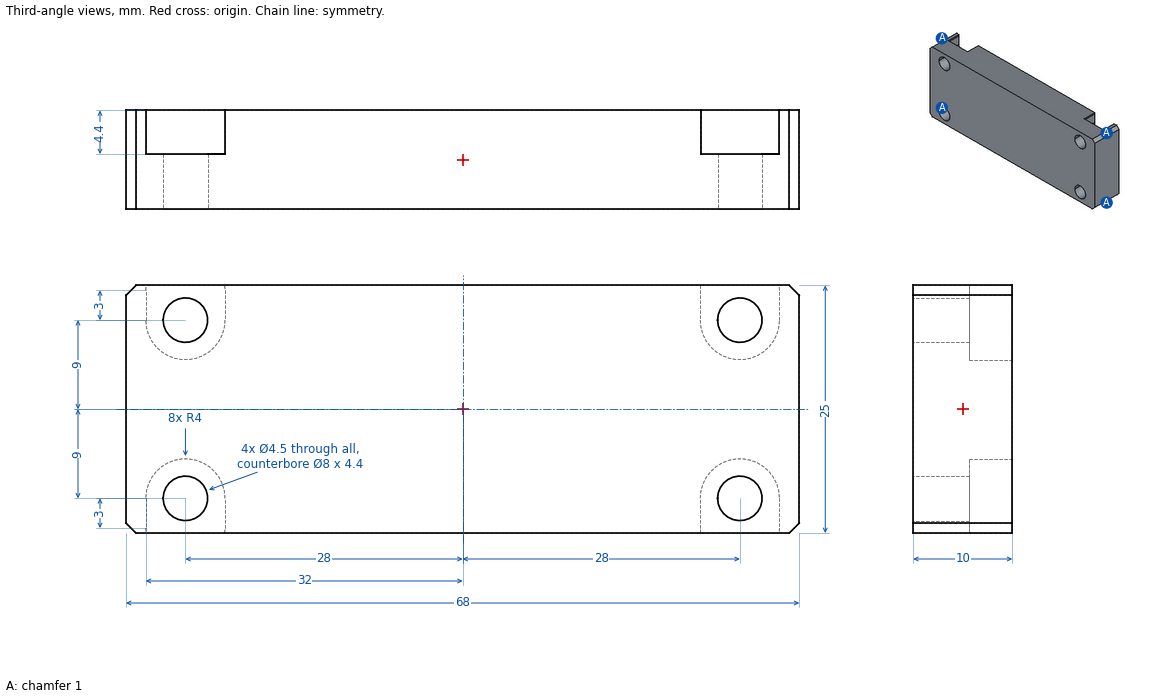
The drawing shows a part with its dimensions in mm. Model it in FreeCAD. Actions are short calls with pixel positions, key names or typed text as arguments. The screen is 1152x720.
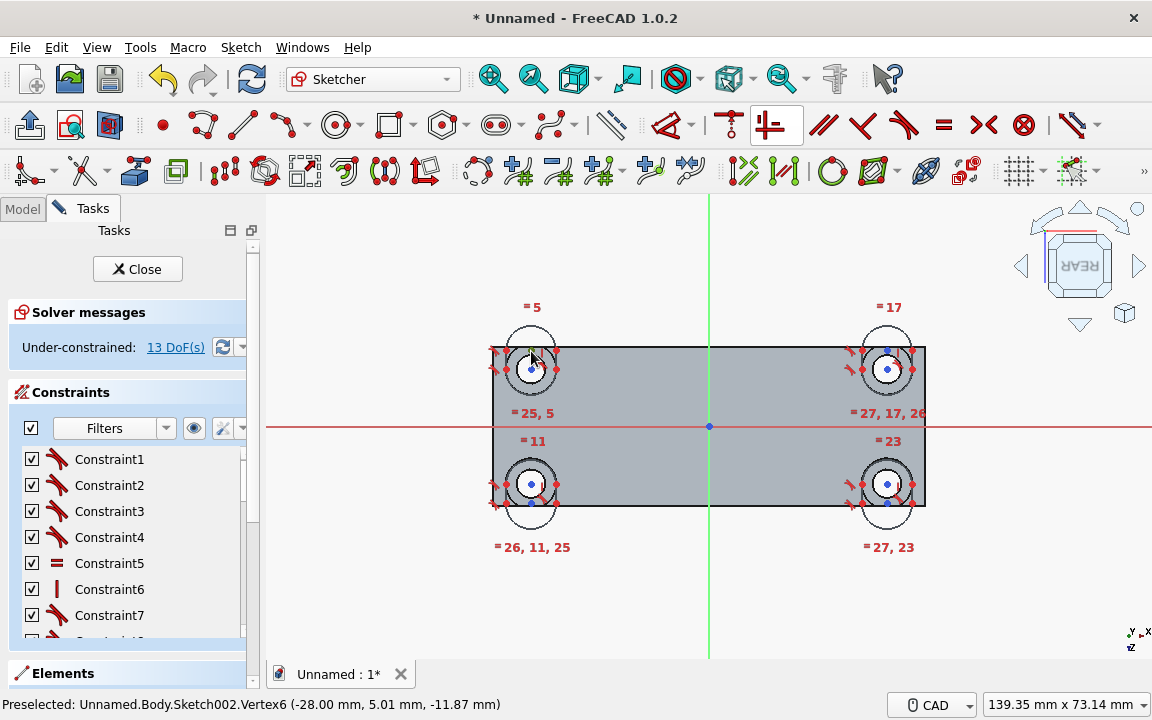
click(531, 504)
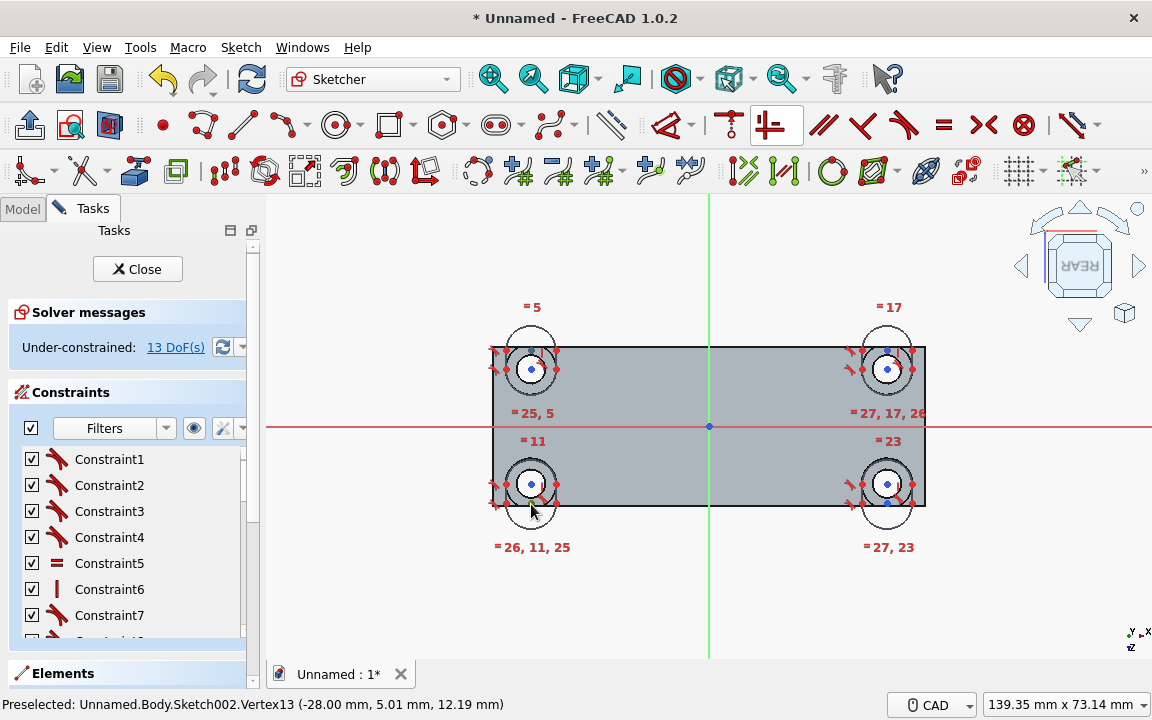
click(344, 426)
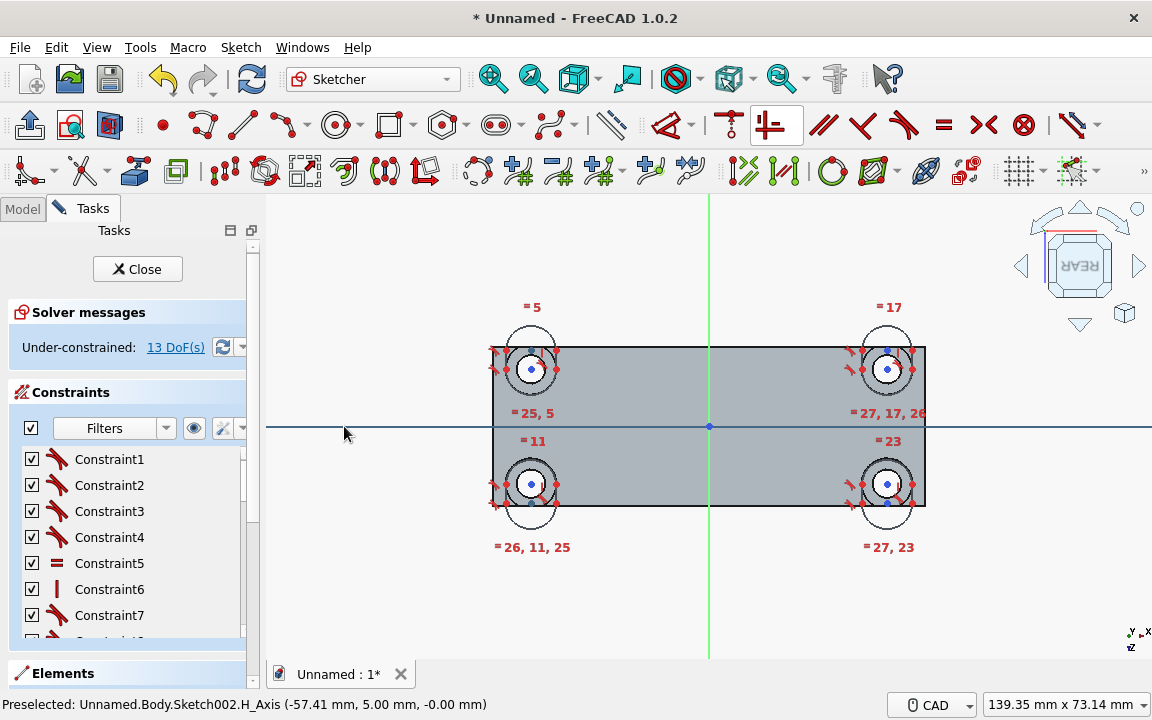
click(984, 126)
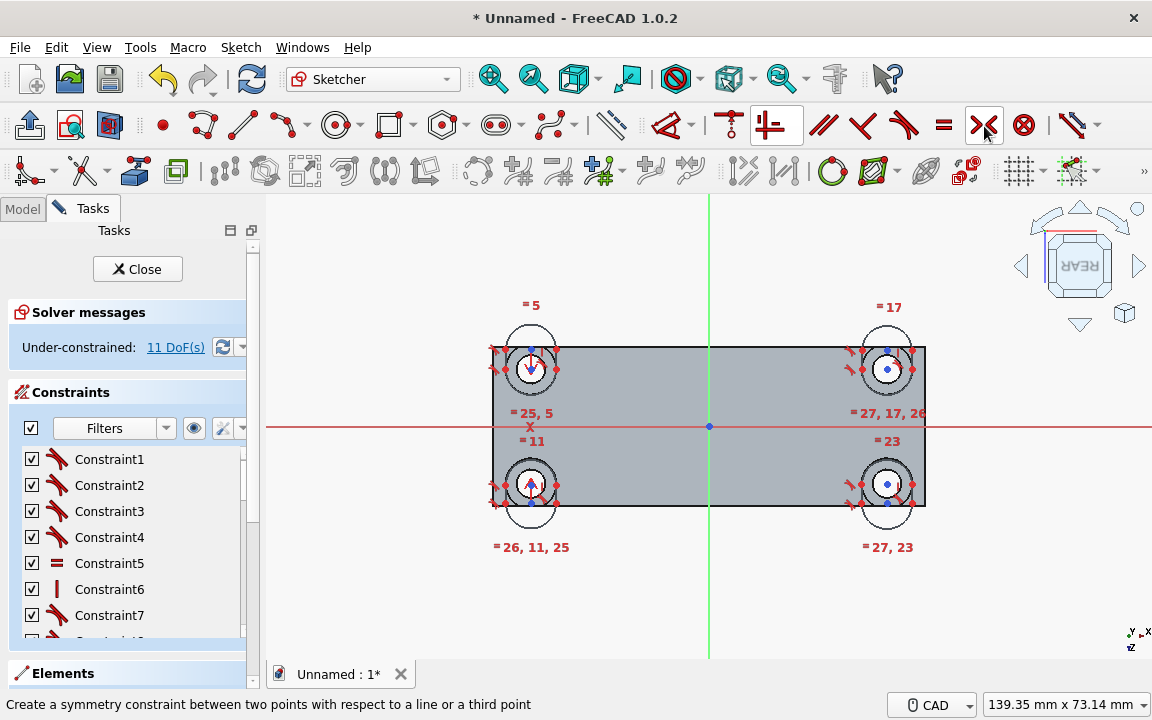
click(531, 370)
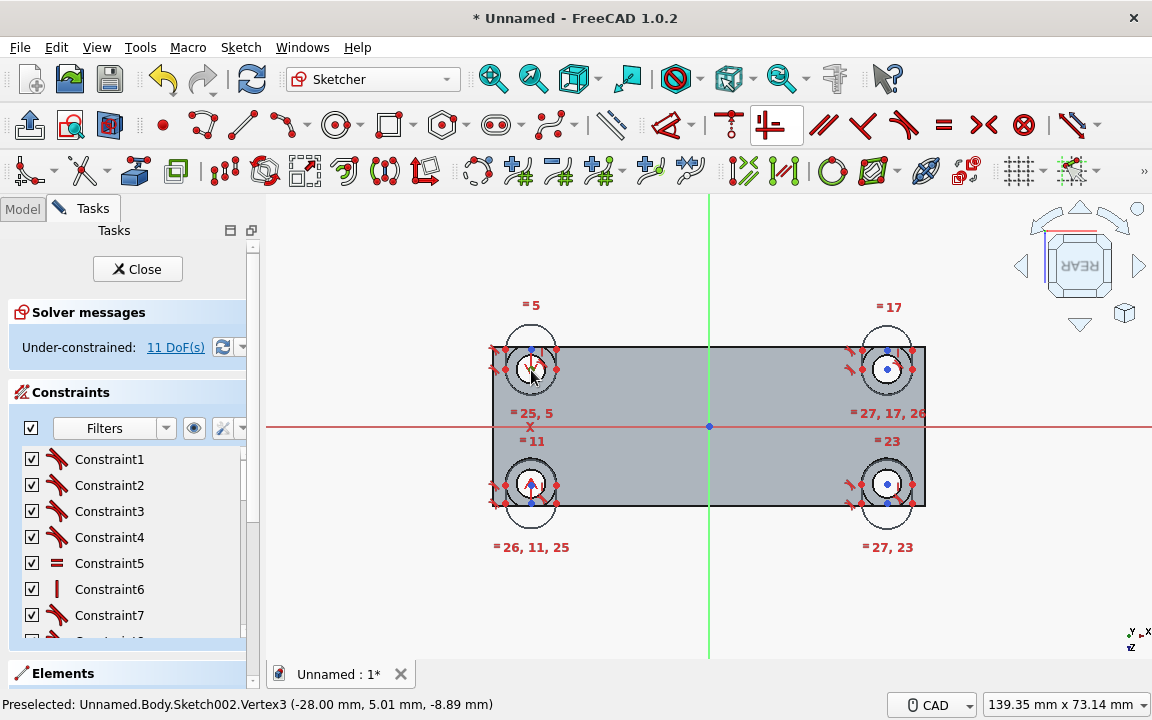
click(887, 370)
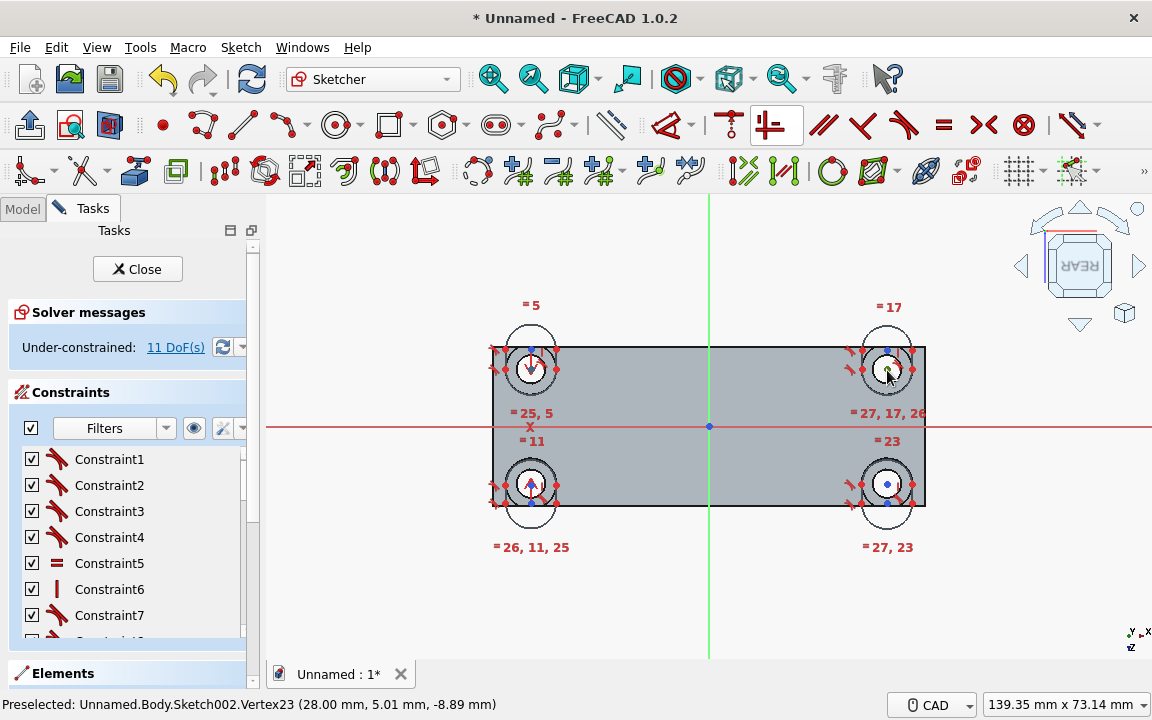
click(709, 602)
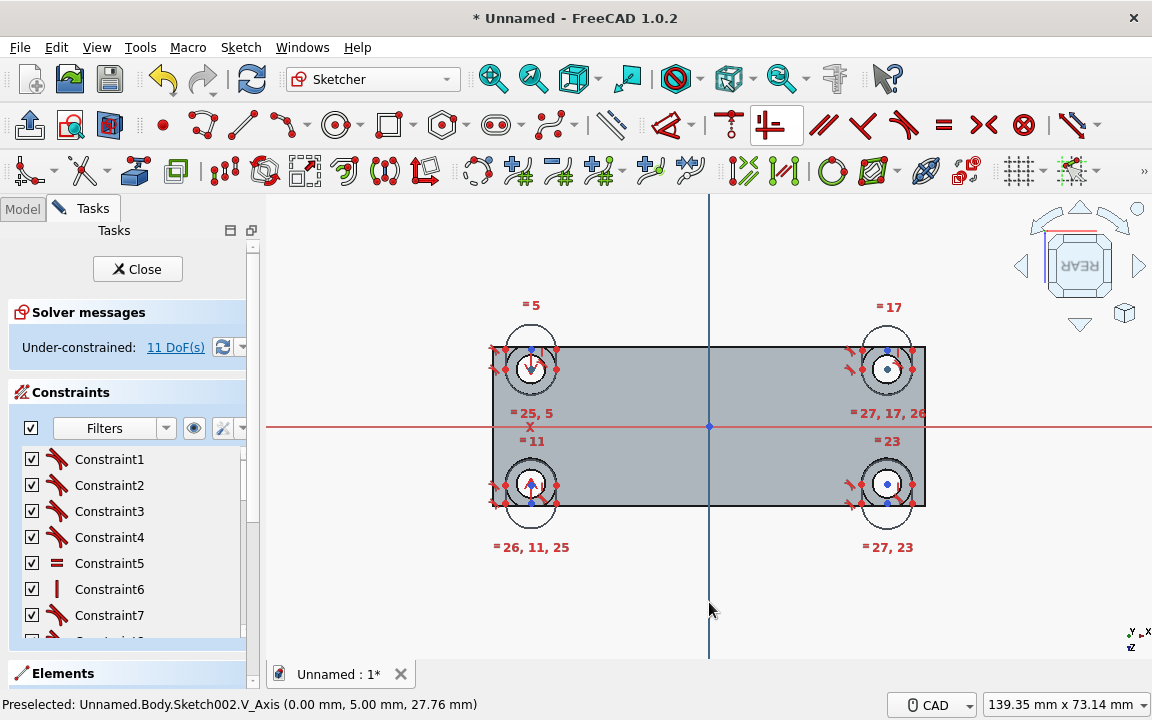
click(984, 126)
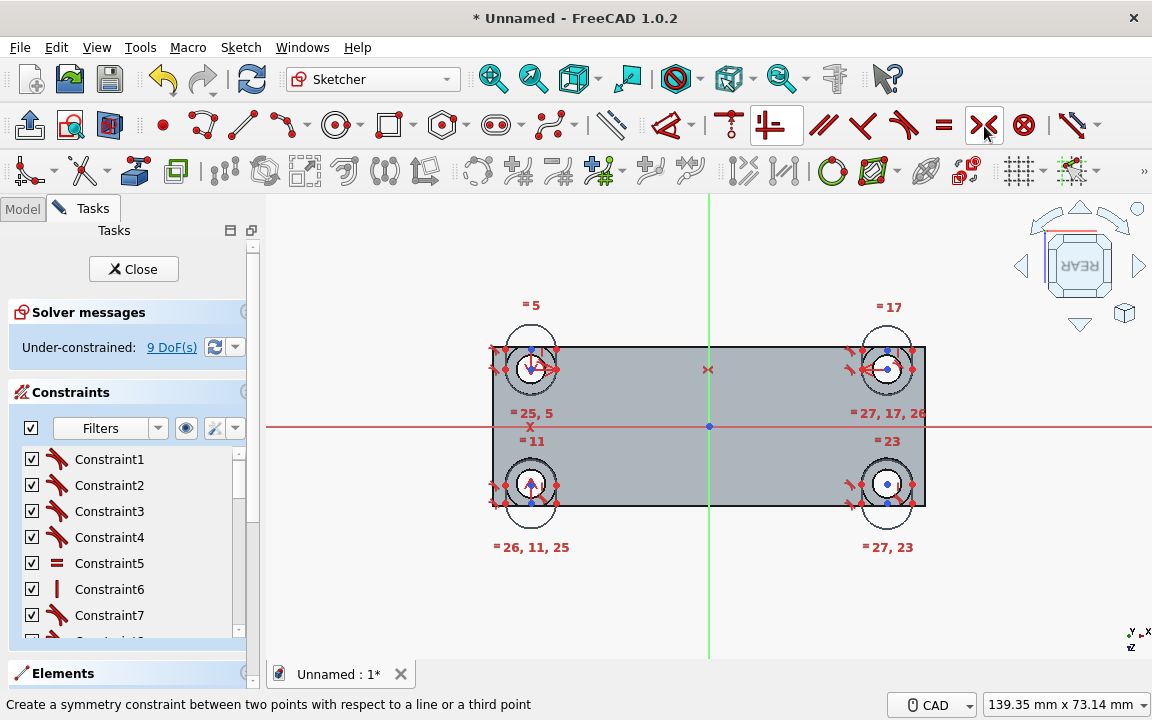
click(531, 503)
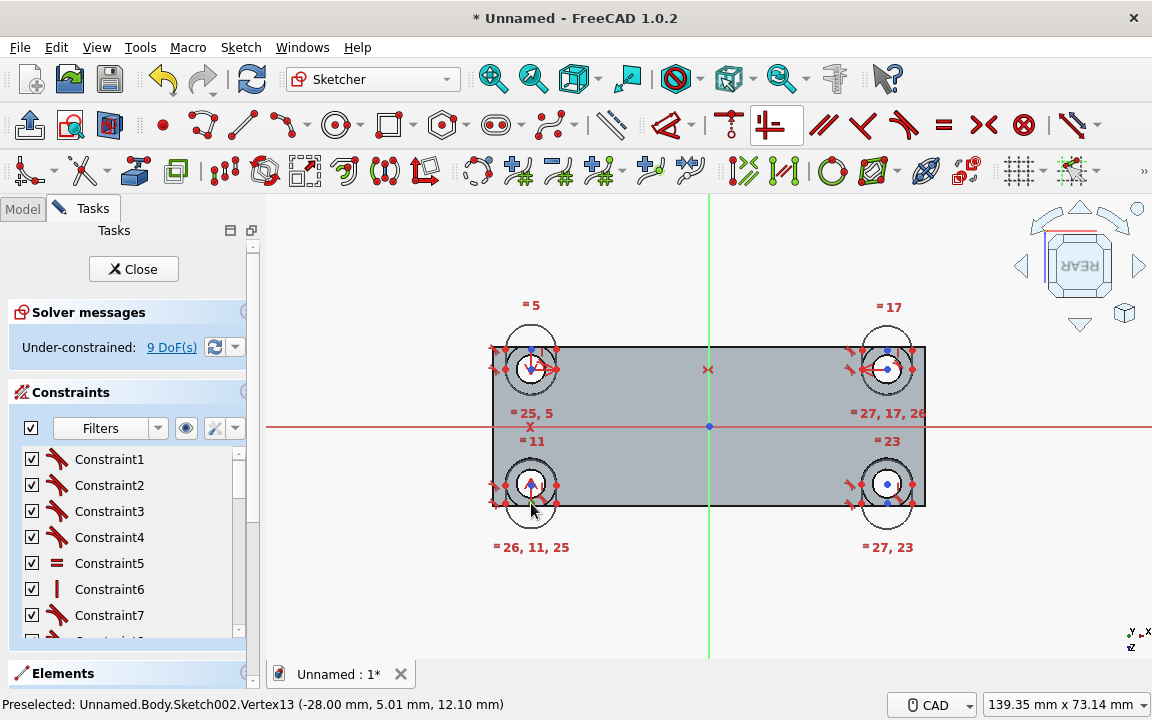
click(887, 504)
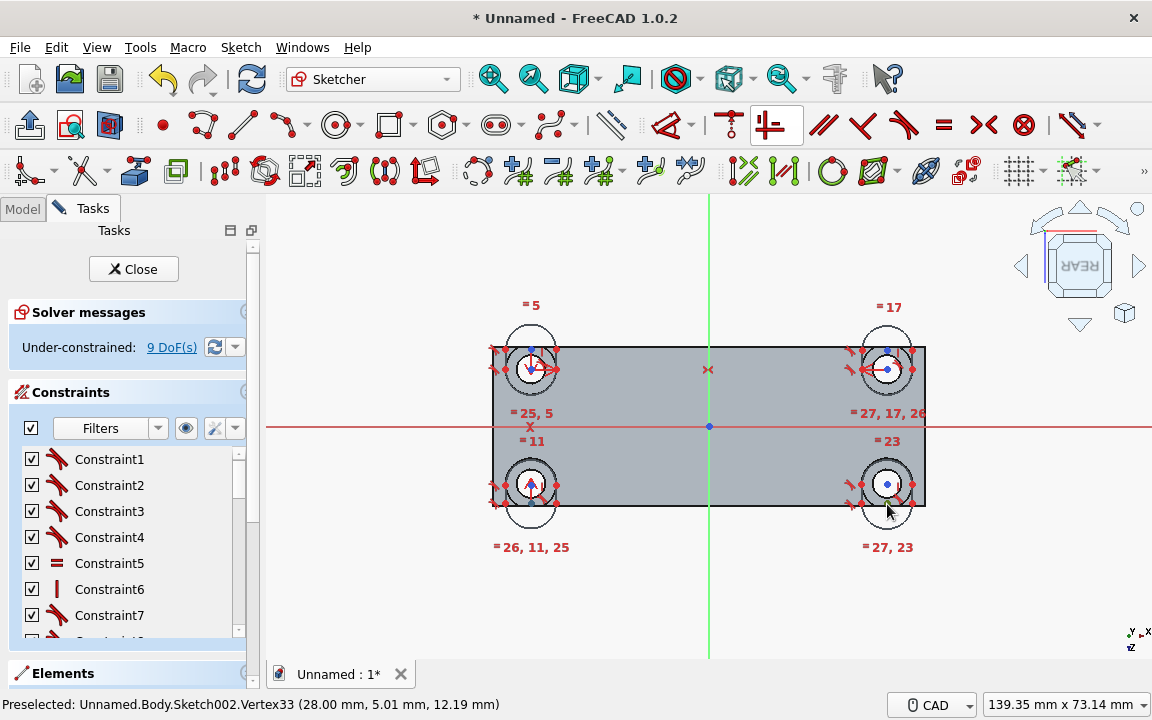
click(709, 602)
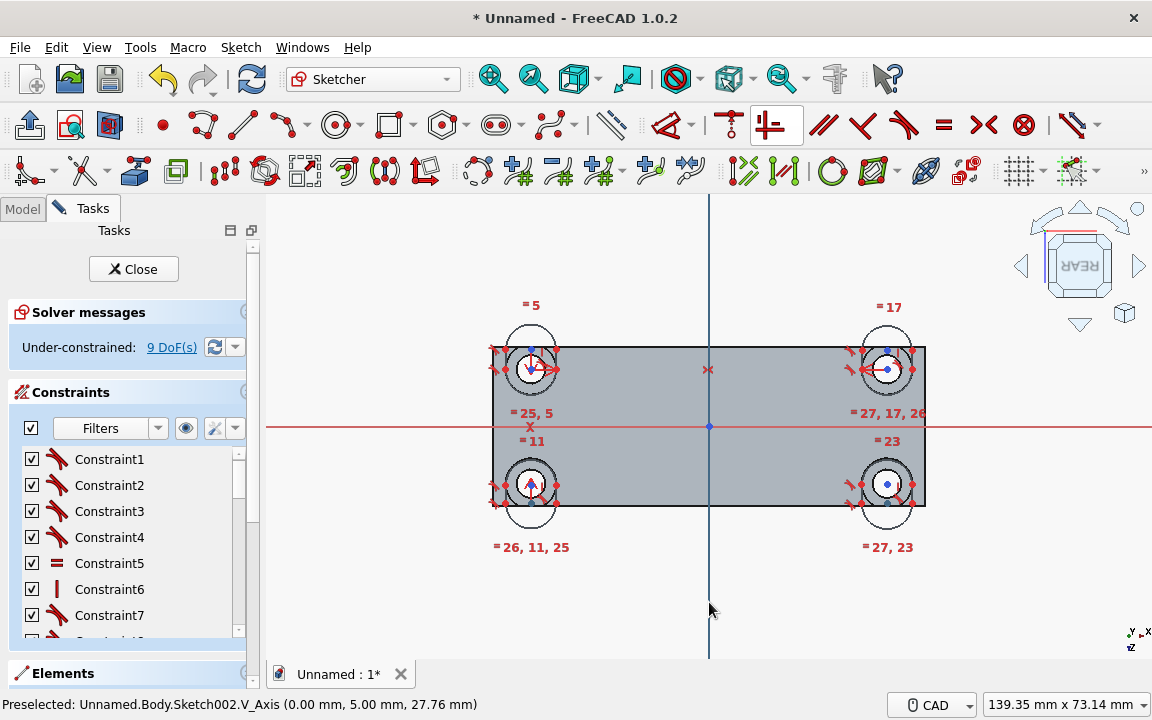
click(984, 126)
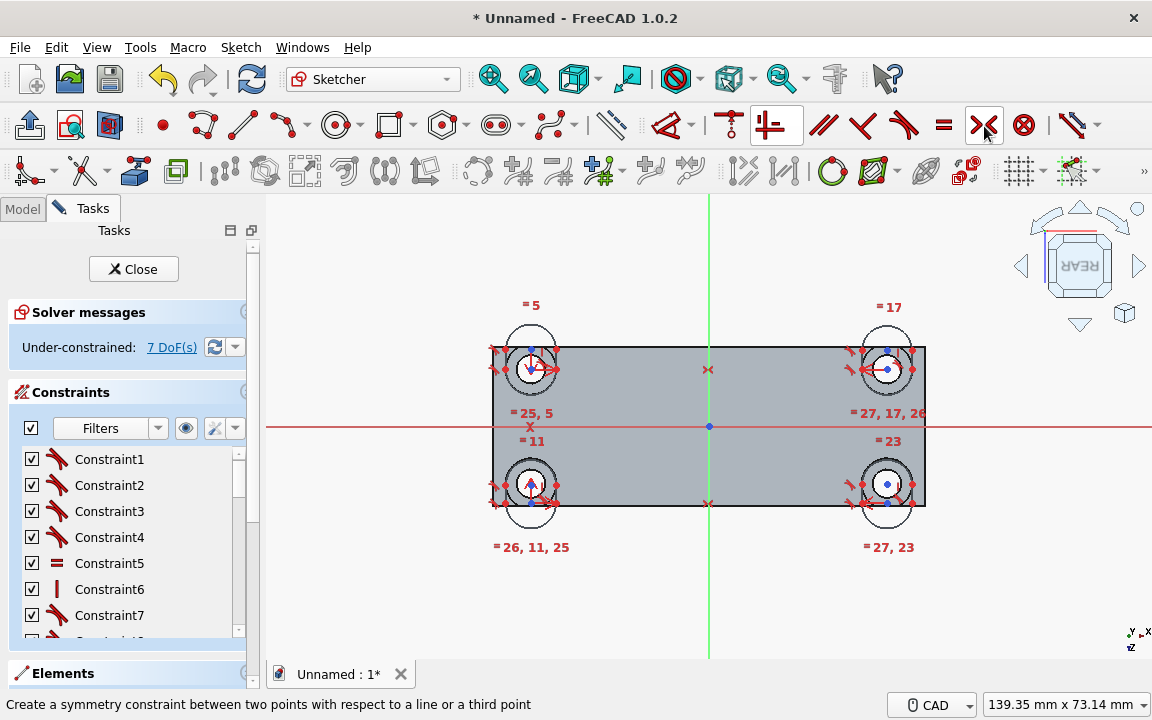
click(666, 126)